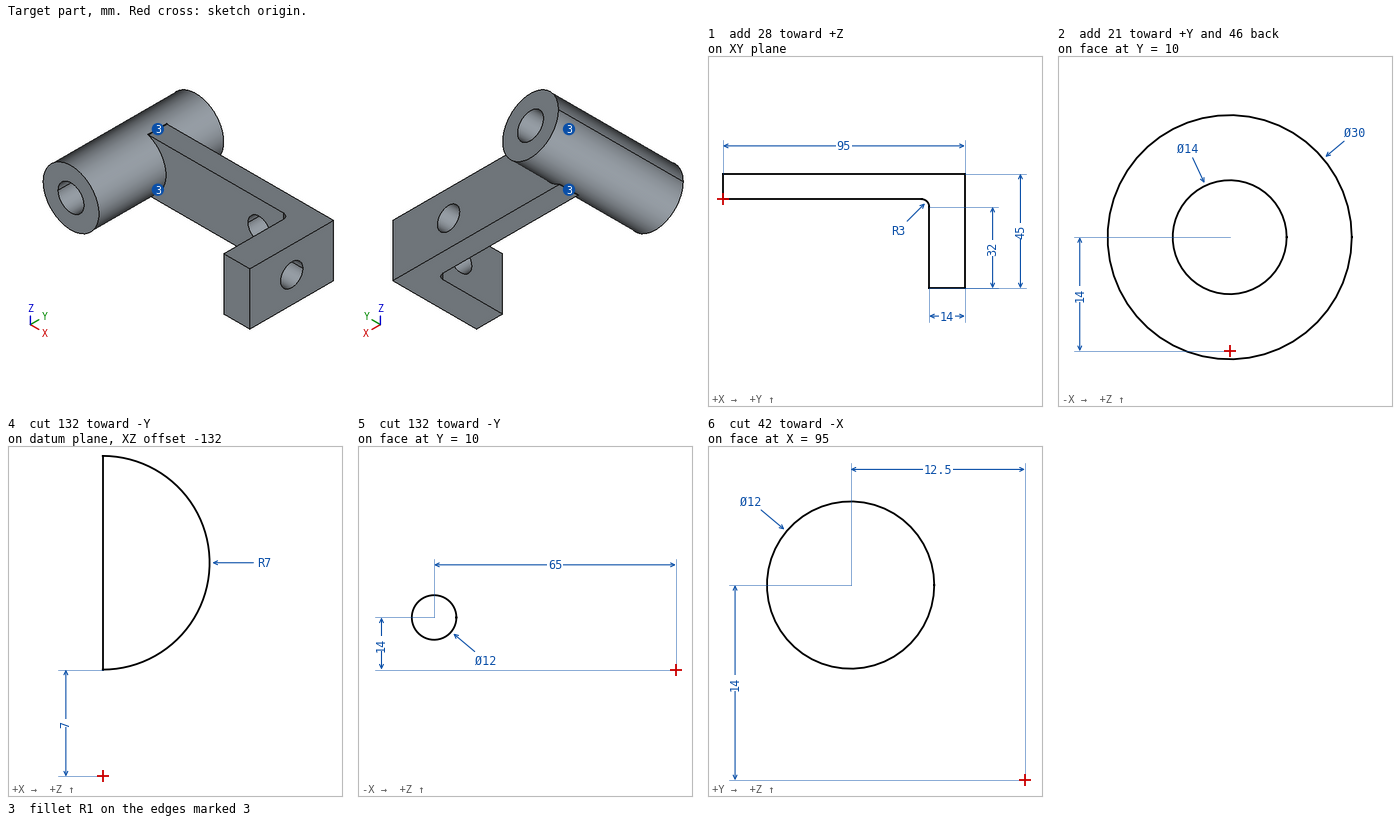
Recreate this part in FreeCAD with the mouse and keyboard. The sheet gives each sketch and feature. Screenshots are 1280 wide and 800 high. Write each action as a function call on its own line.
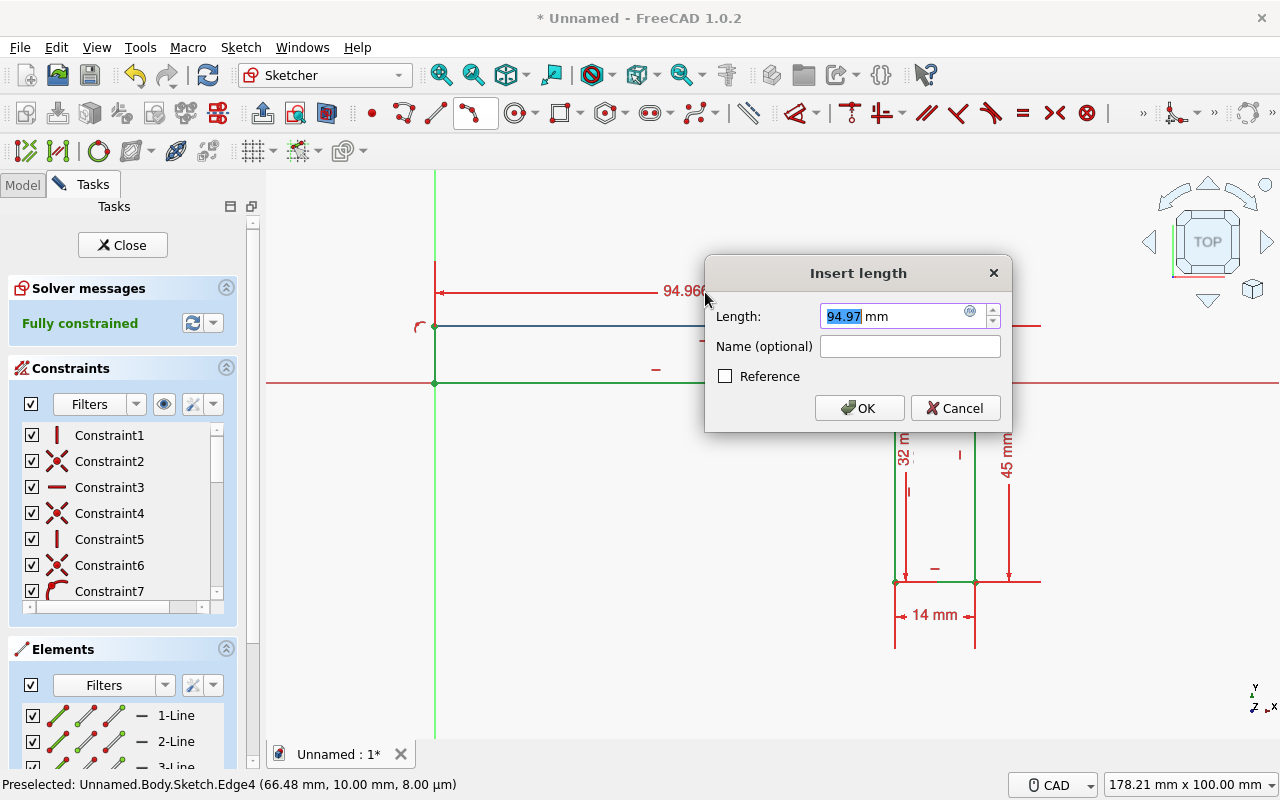
text(95)
key(Return)
key(Escape)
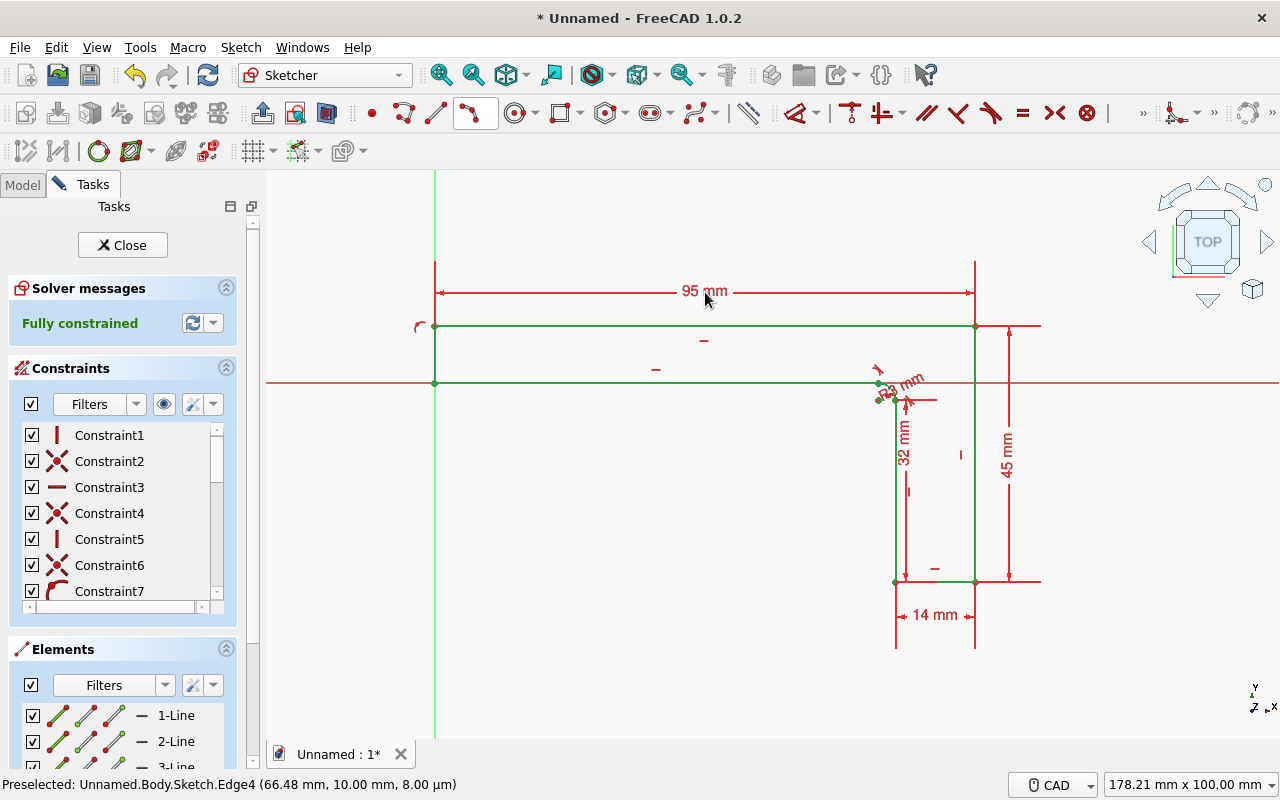
click(123, 245)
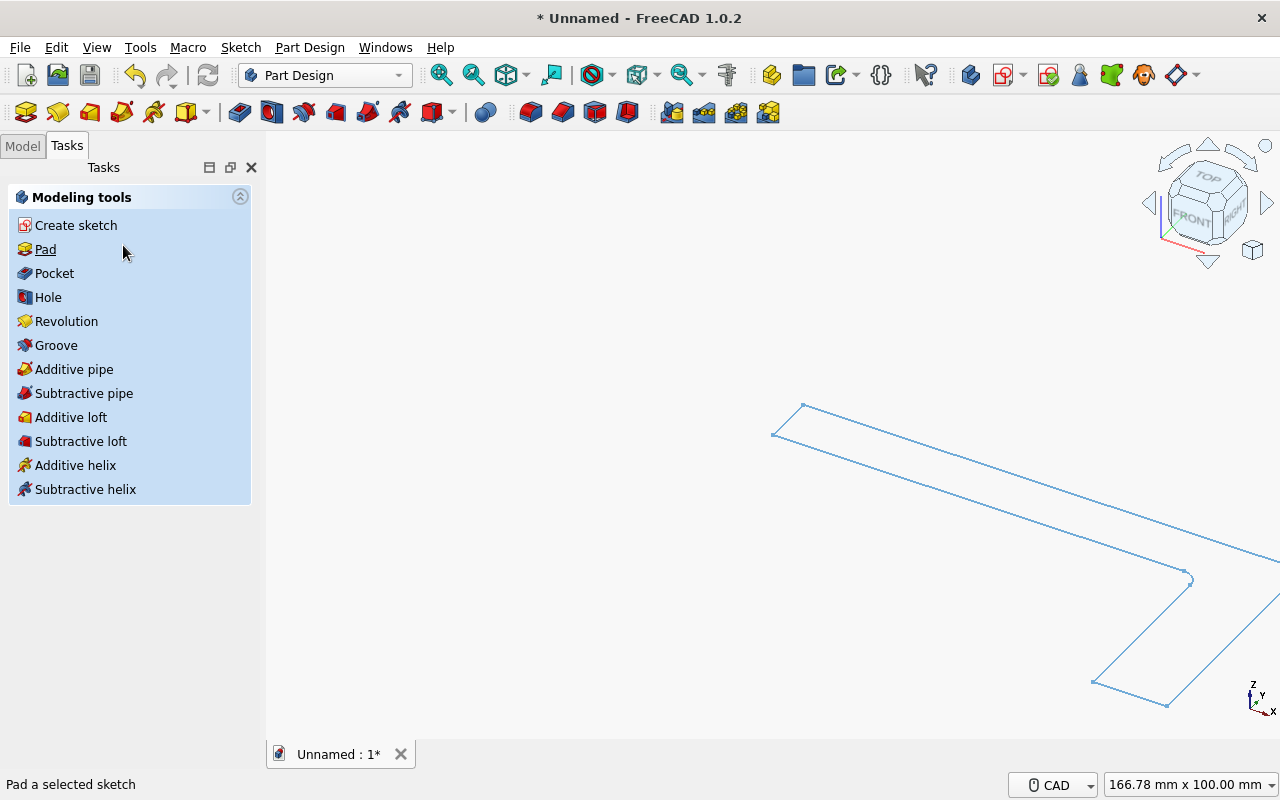
click(26, 112)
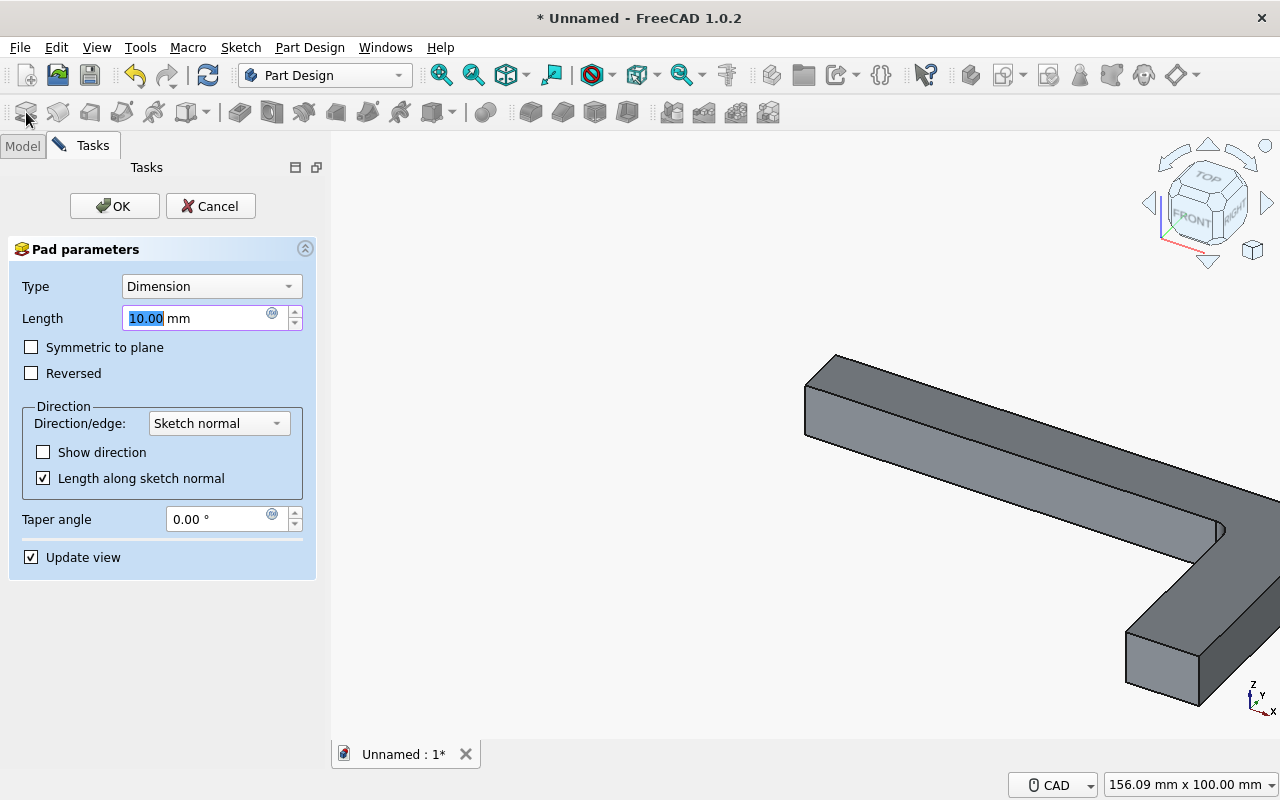
text(28)
key(Tab)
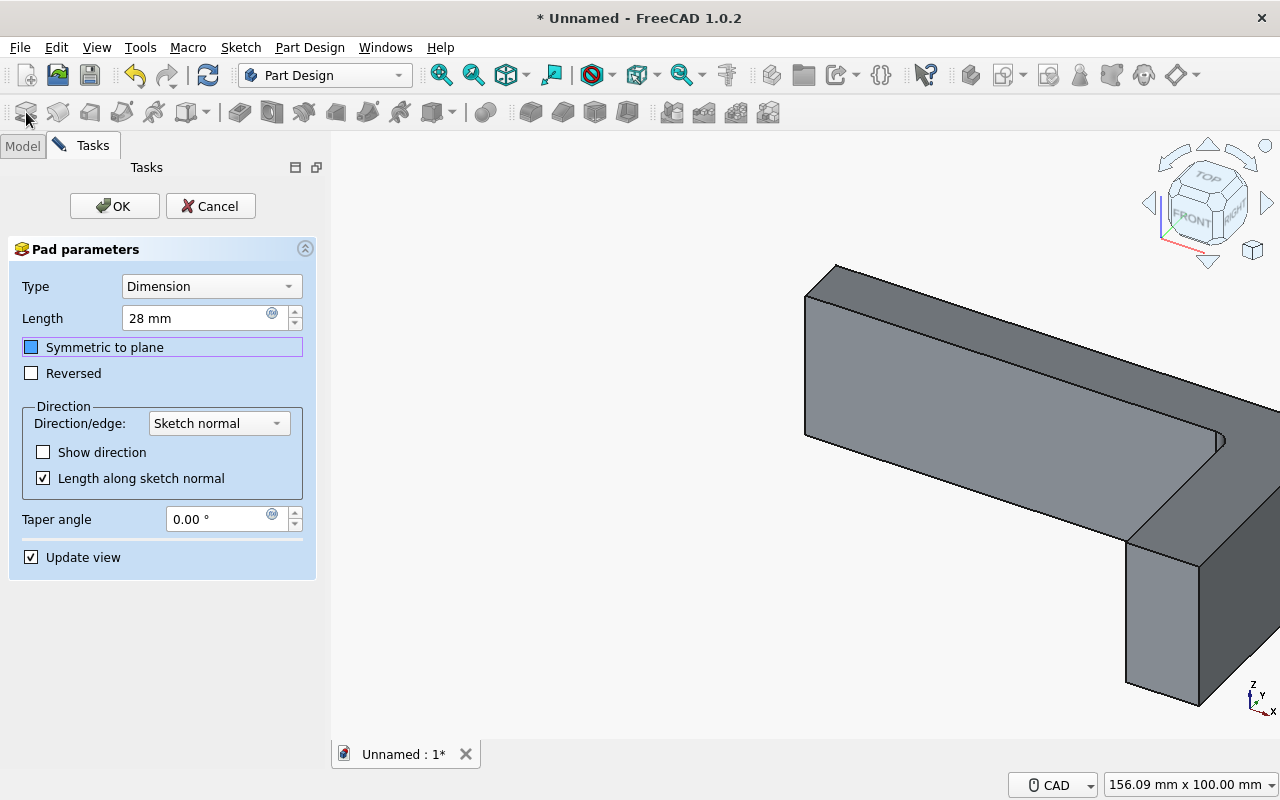
click(115, 206)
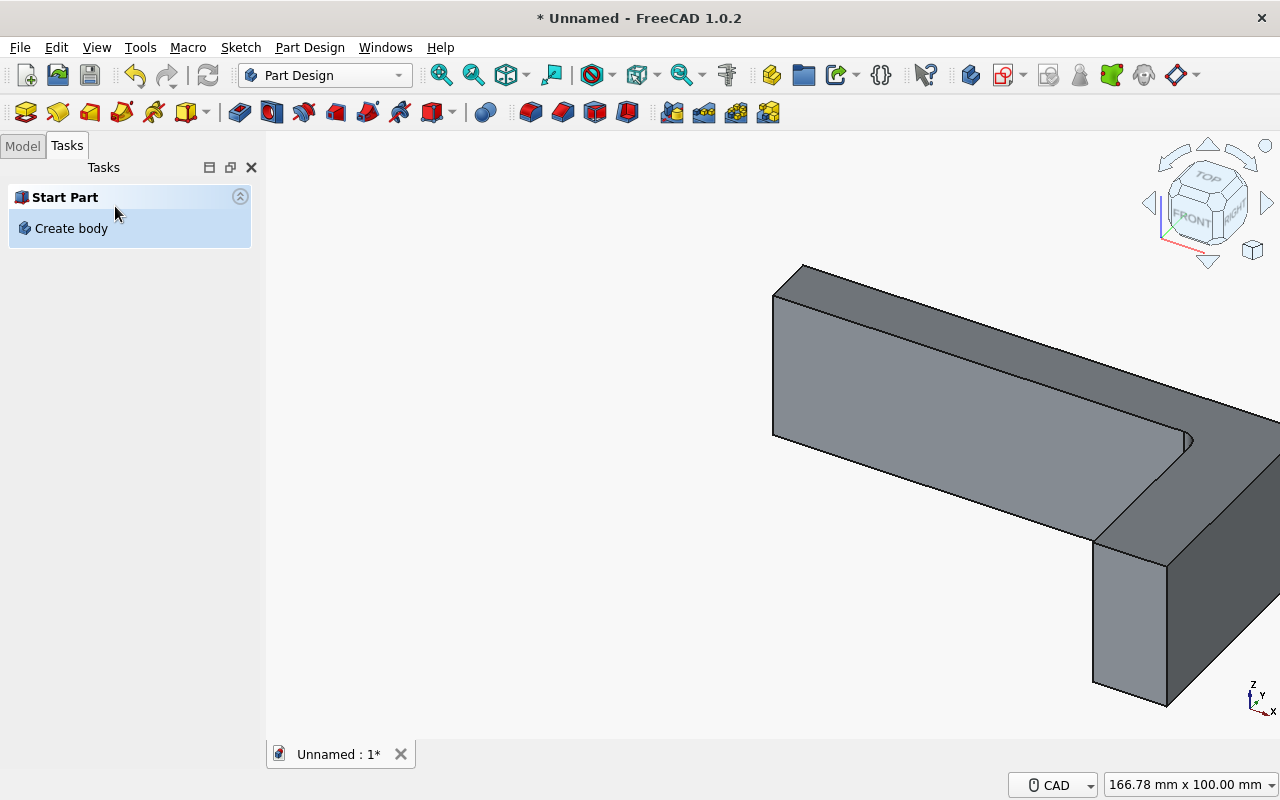
click(442, 76)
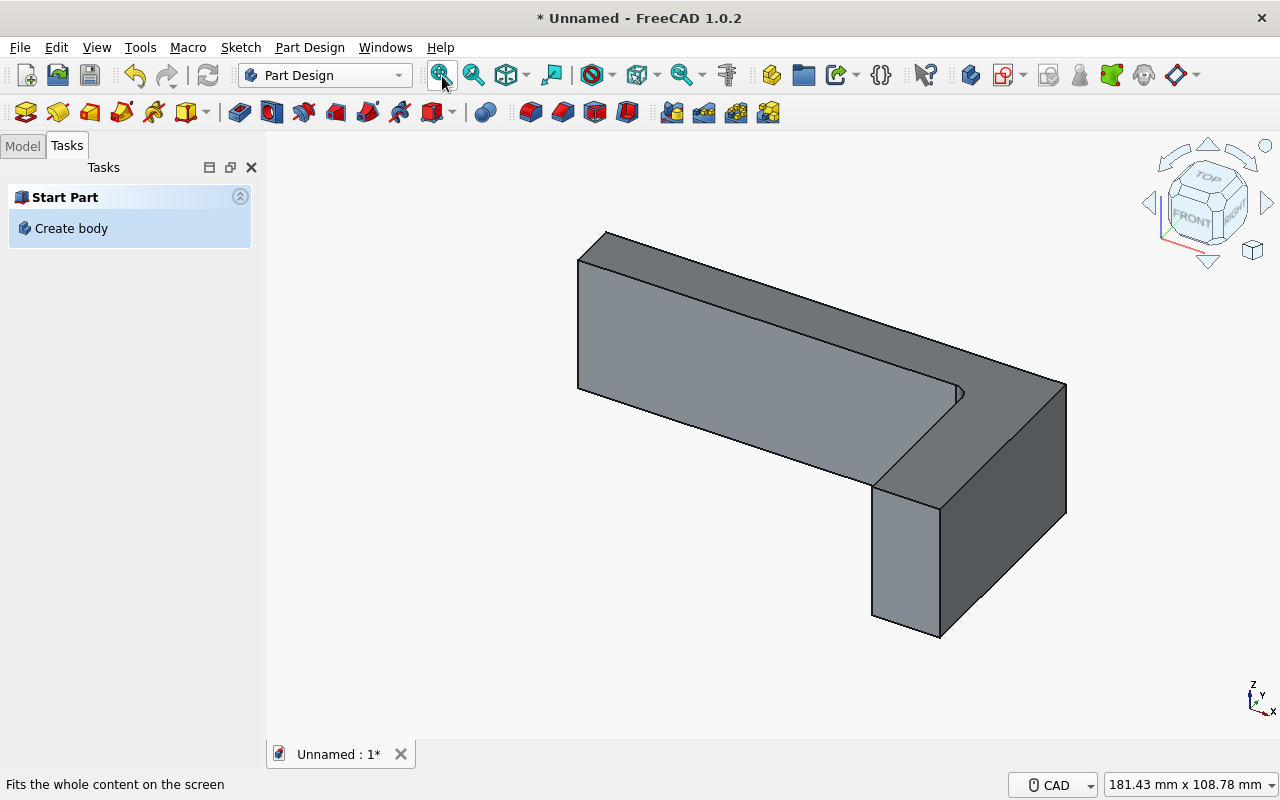
key(4)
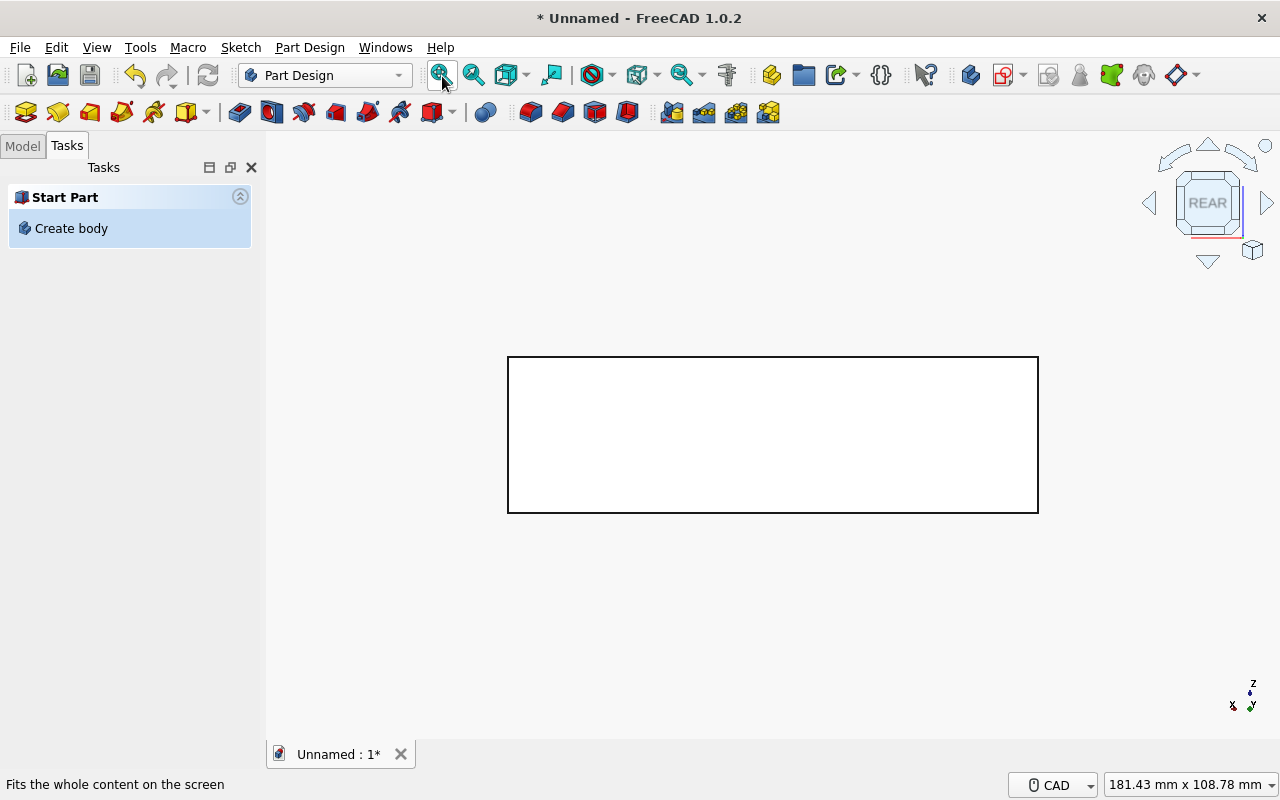
click(621, 434)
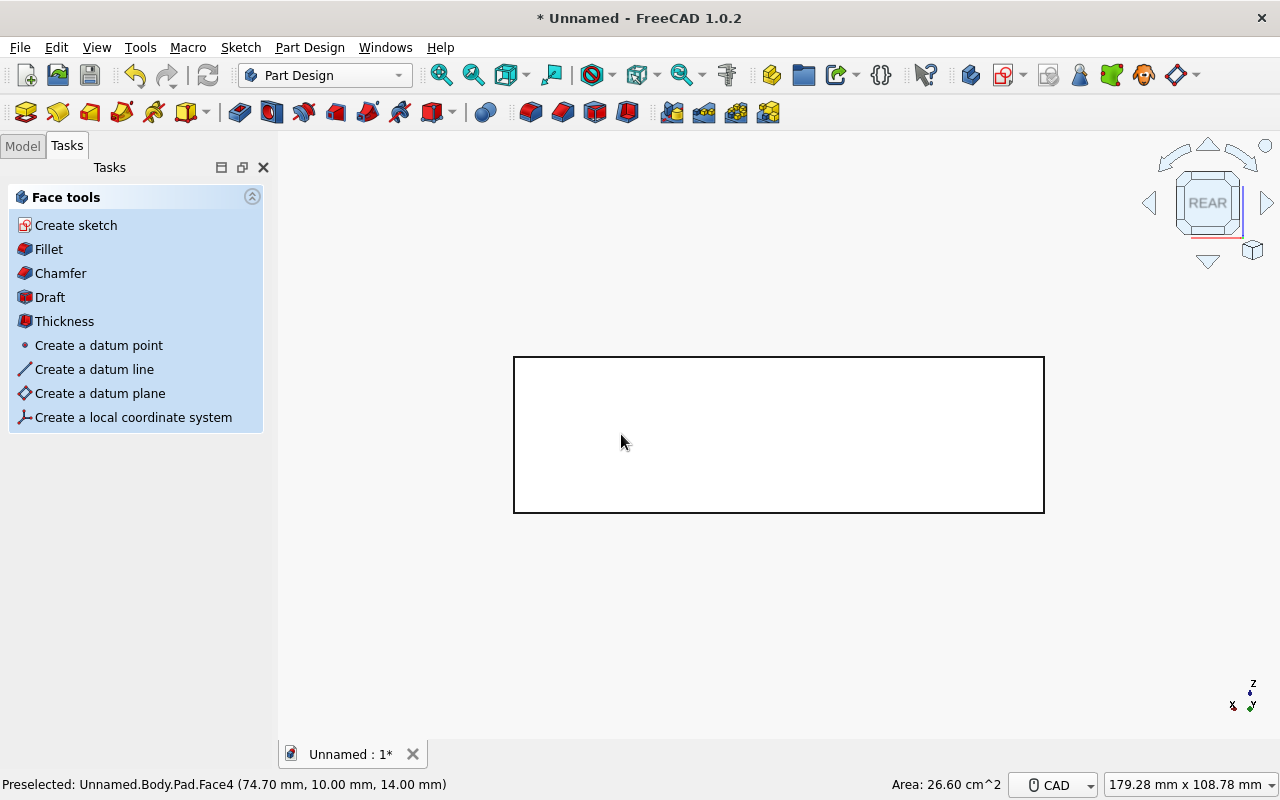
click(1004, 76)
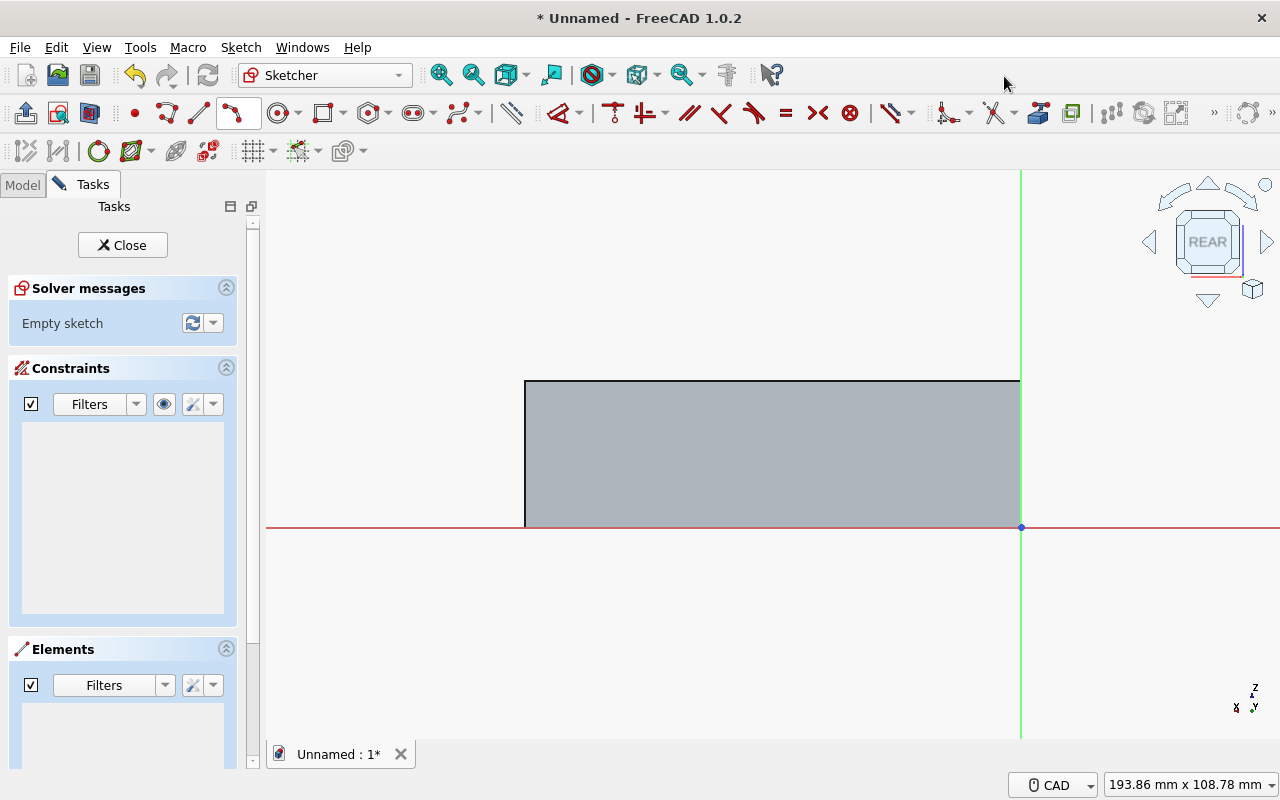
scroll(1115, 454, up, 4)